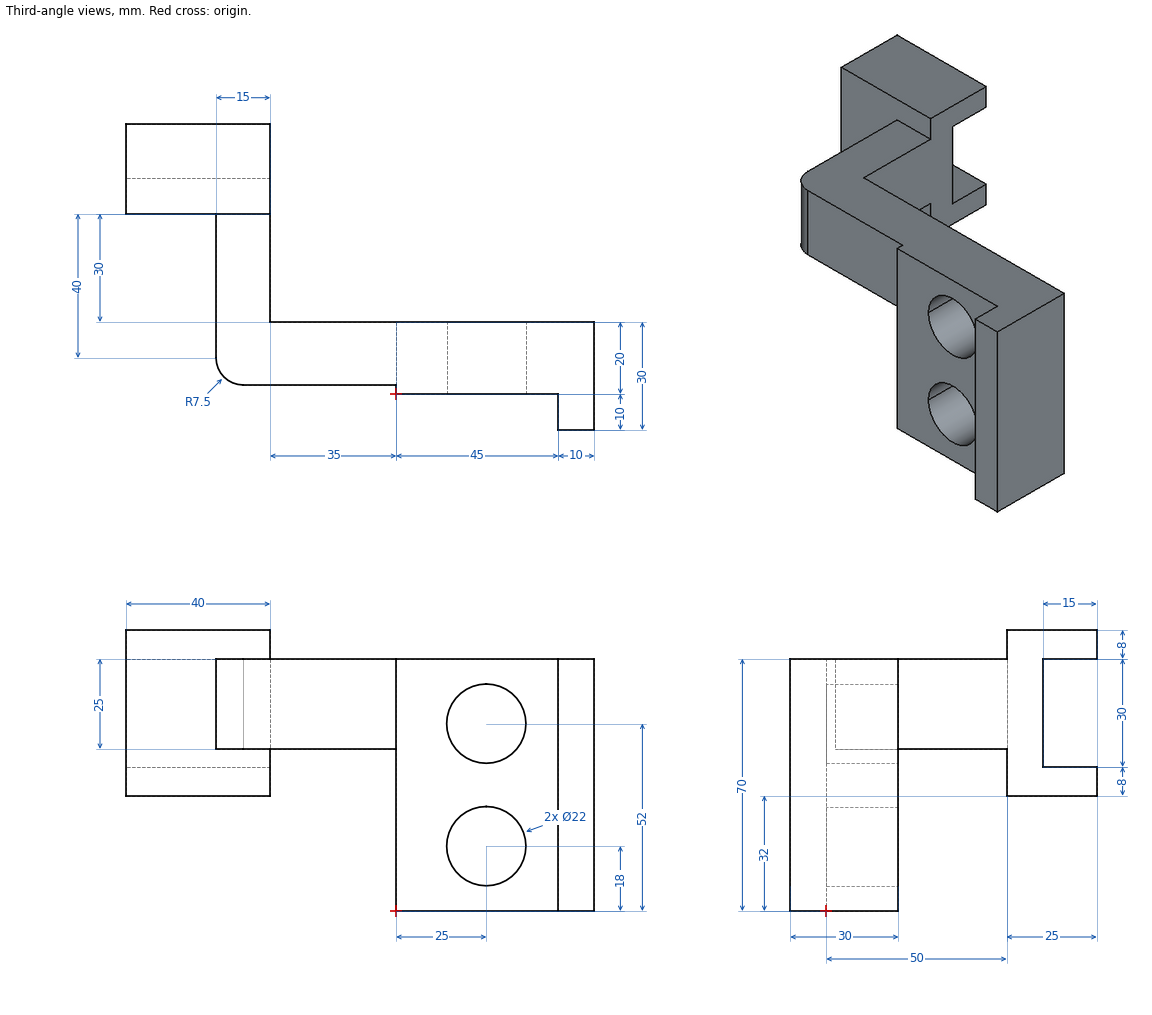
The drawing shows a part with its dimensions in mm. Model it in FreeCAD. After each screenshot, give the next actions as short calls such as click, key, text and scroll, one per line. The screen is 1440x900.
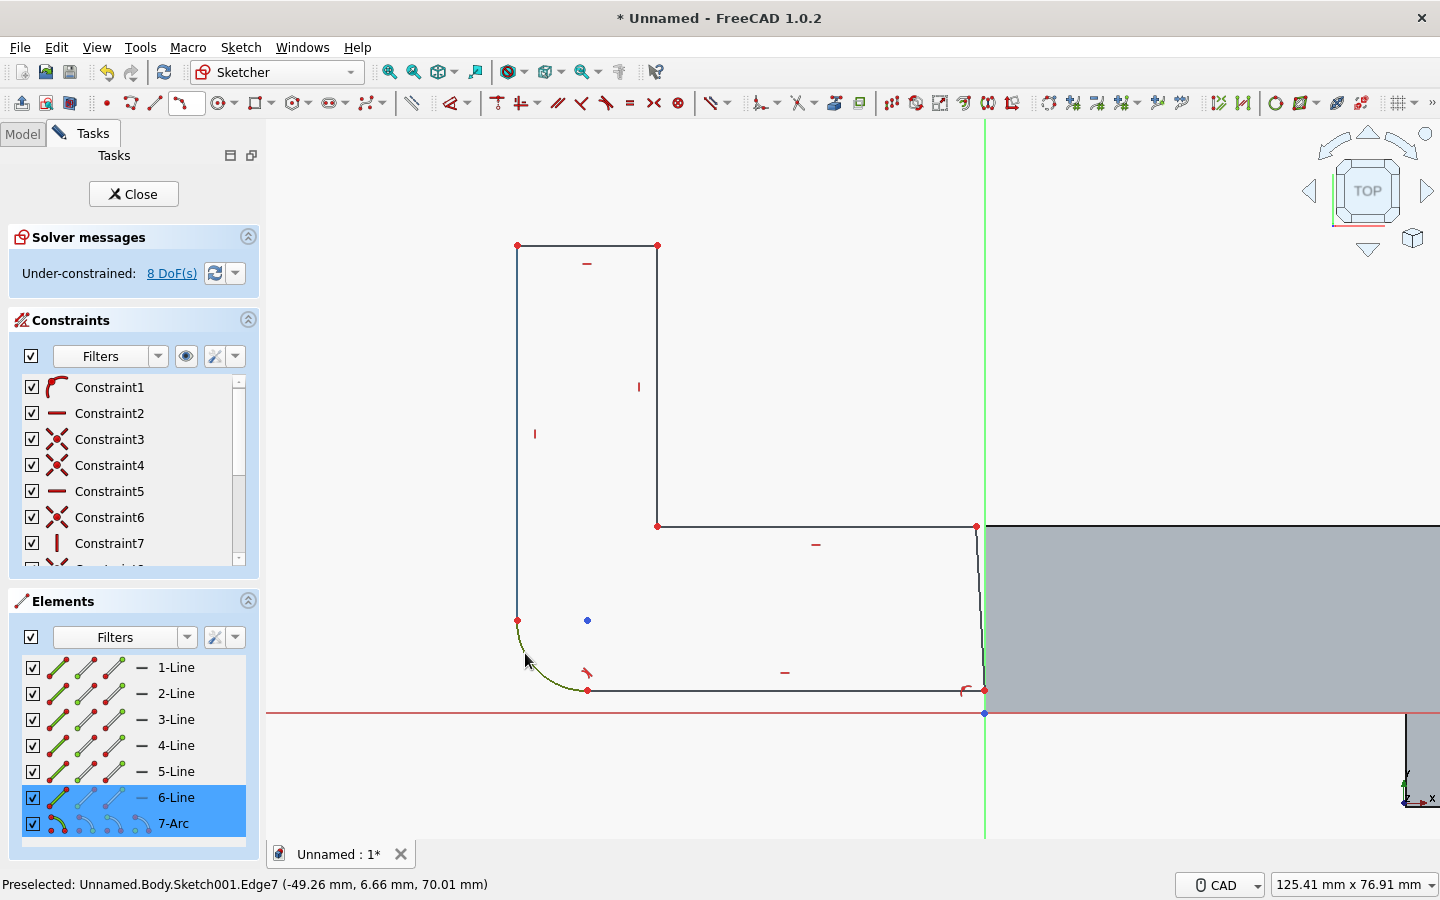
click(606, 104)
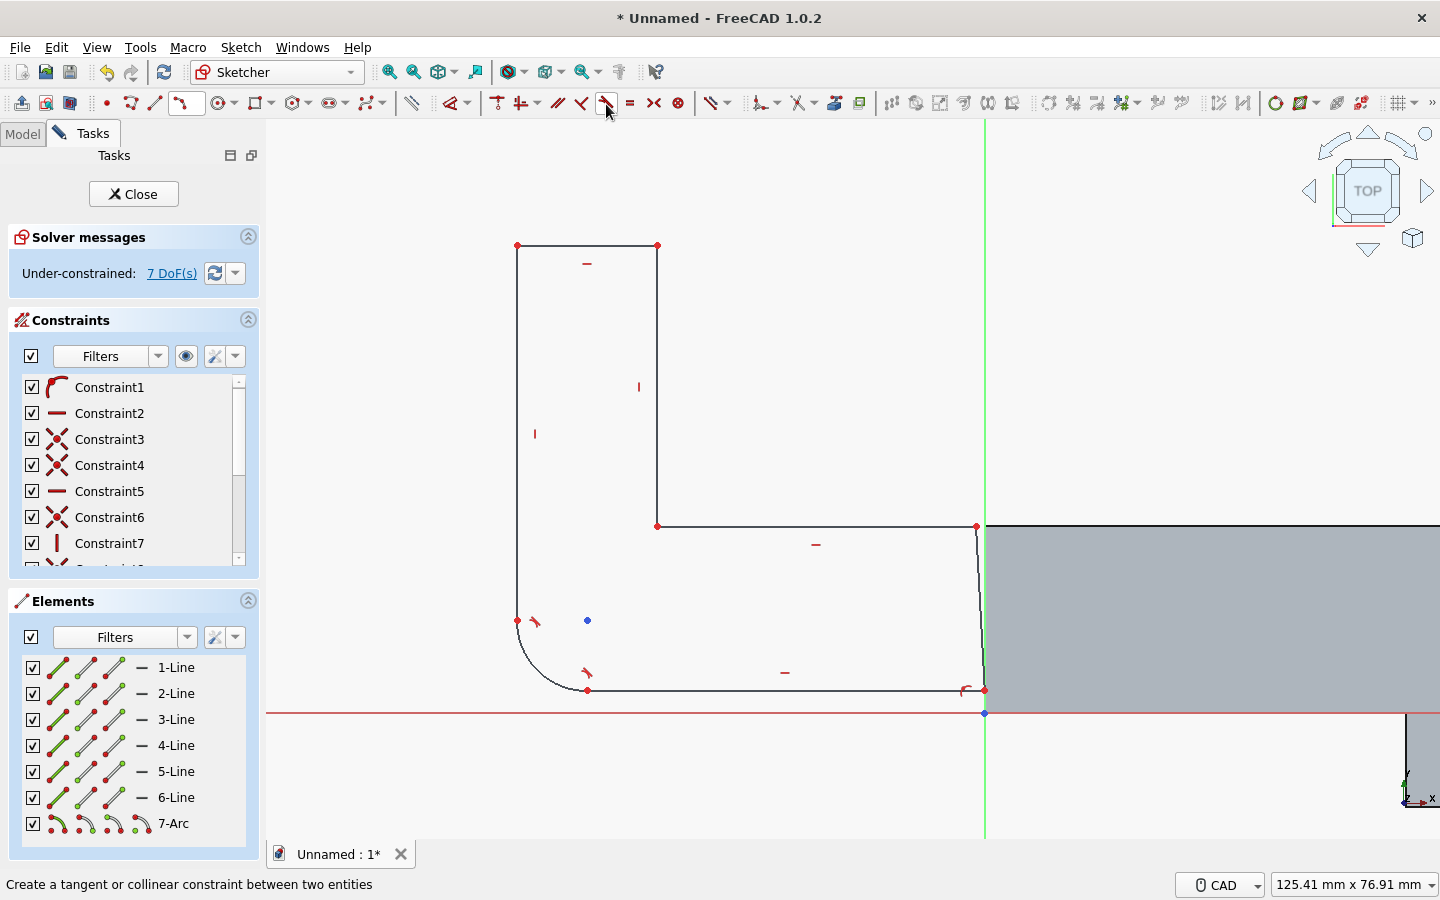
click(982, 642)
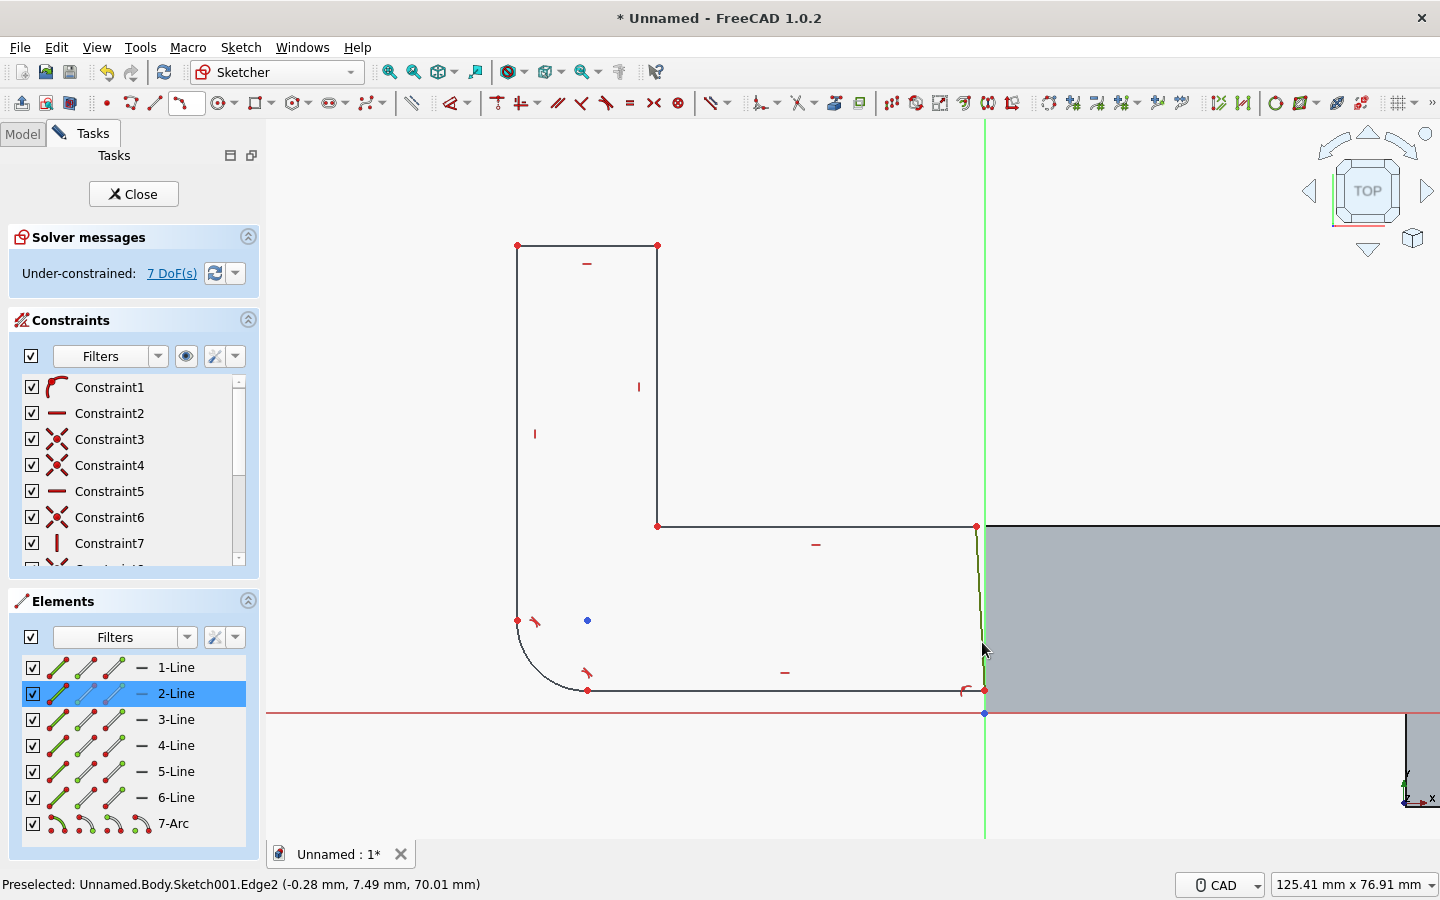
click(540, 104)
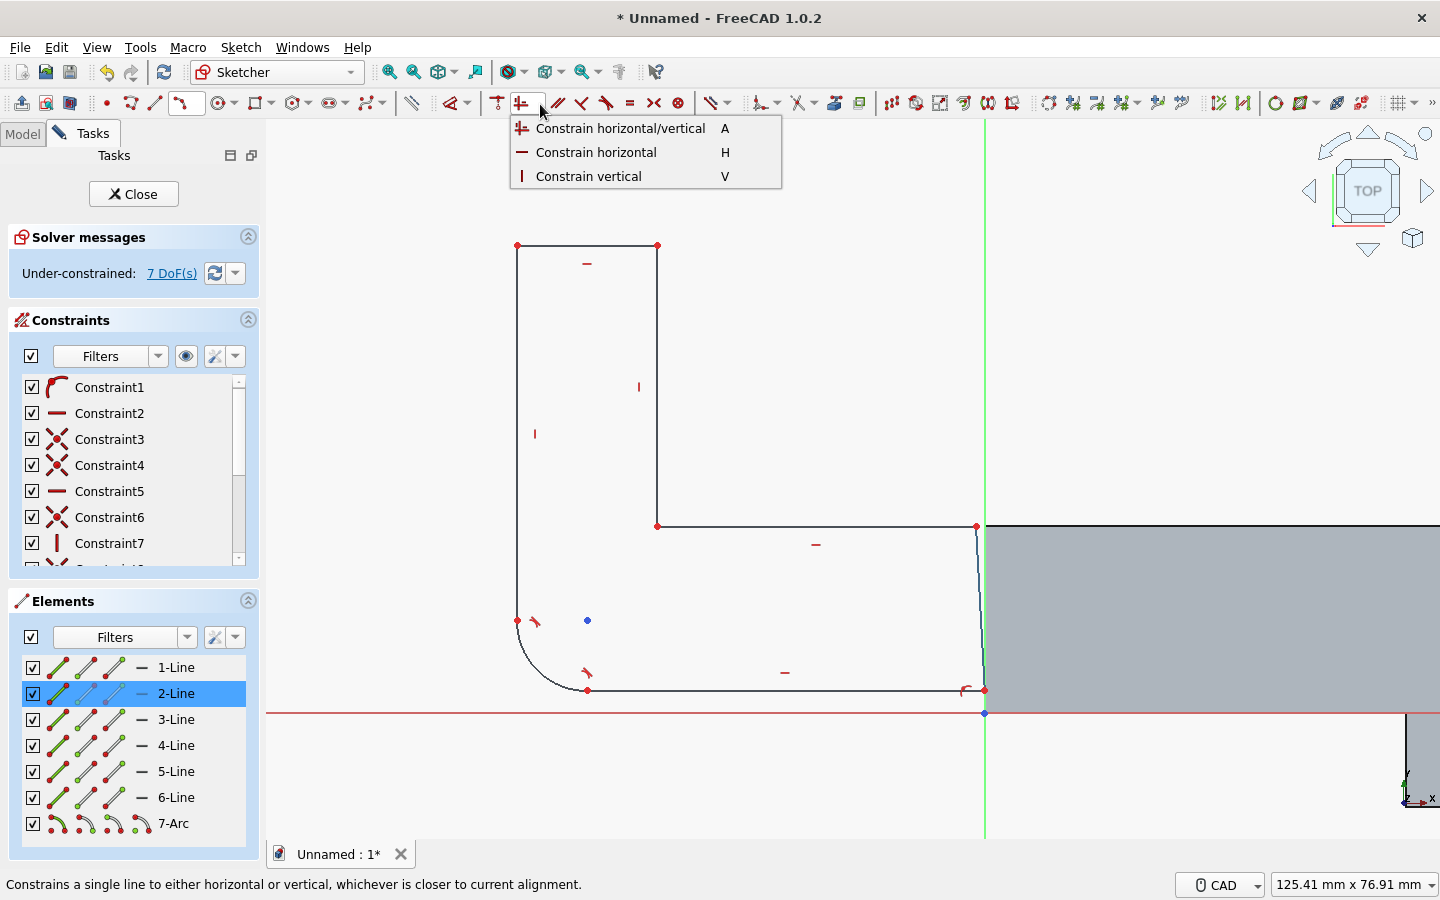
click(646, 176)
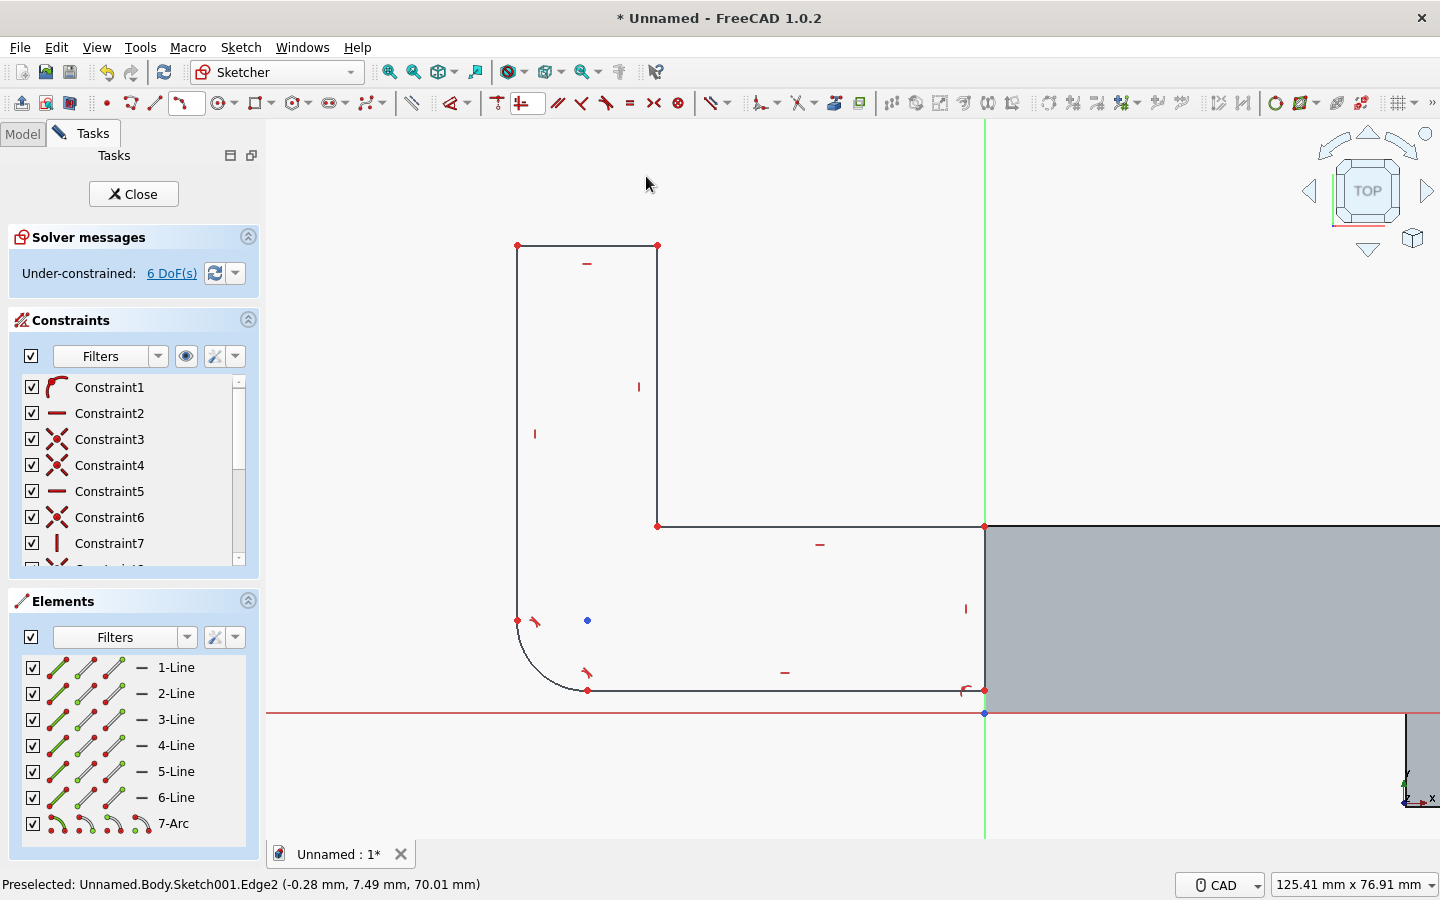
click(450, 104)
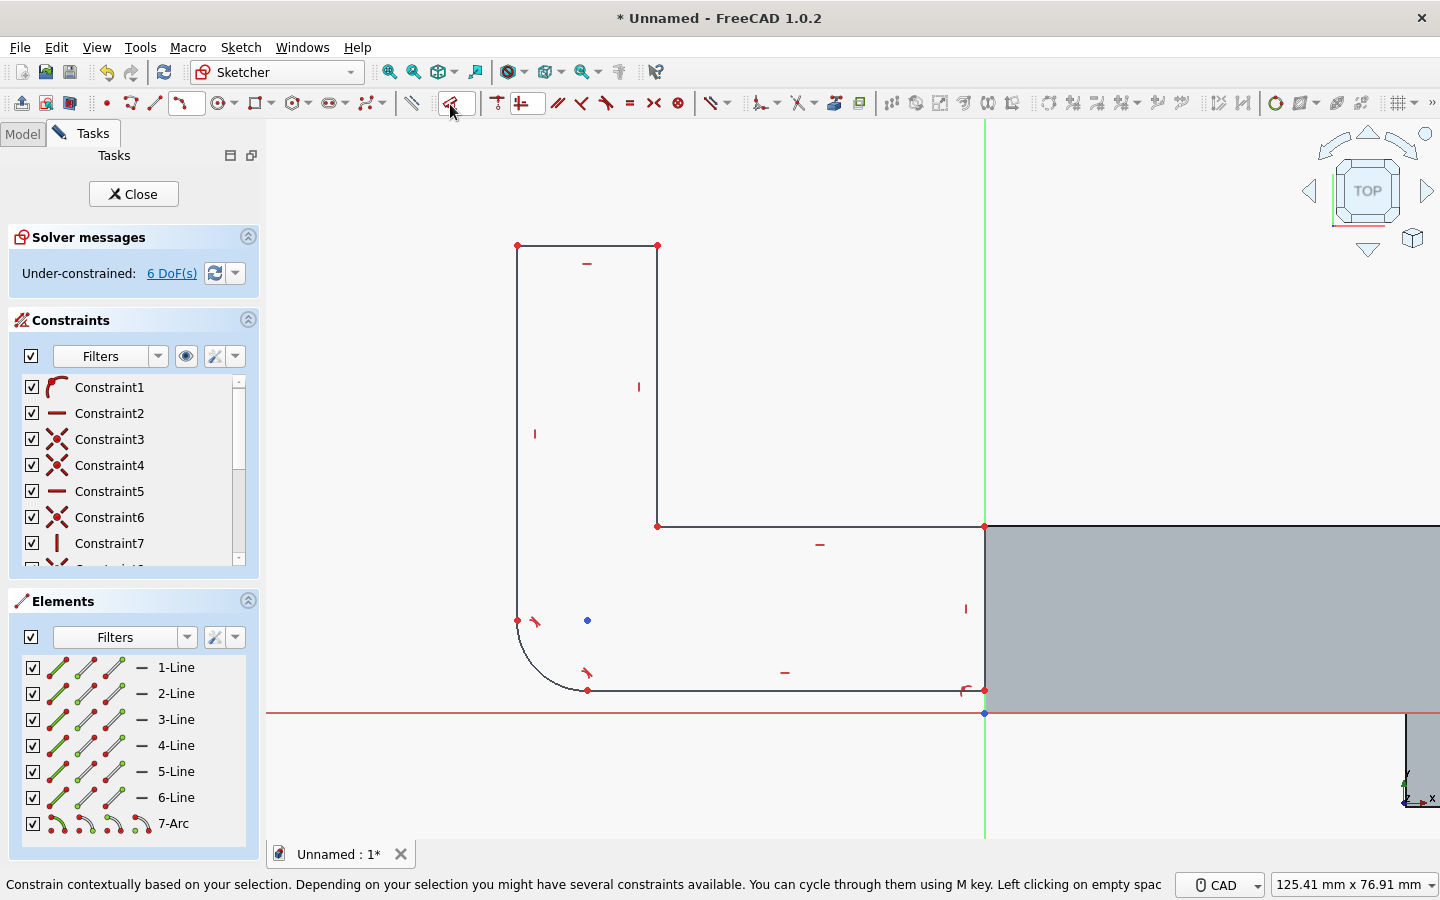
click(525, 653)
click(497, 668)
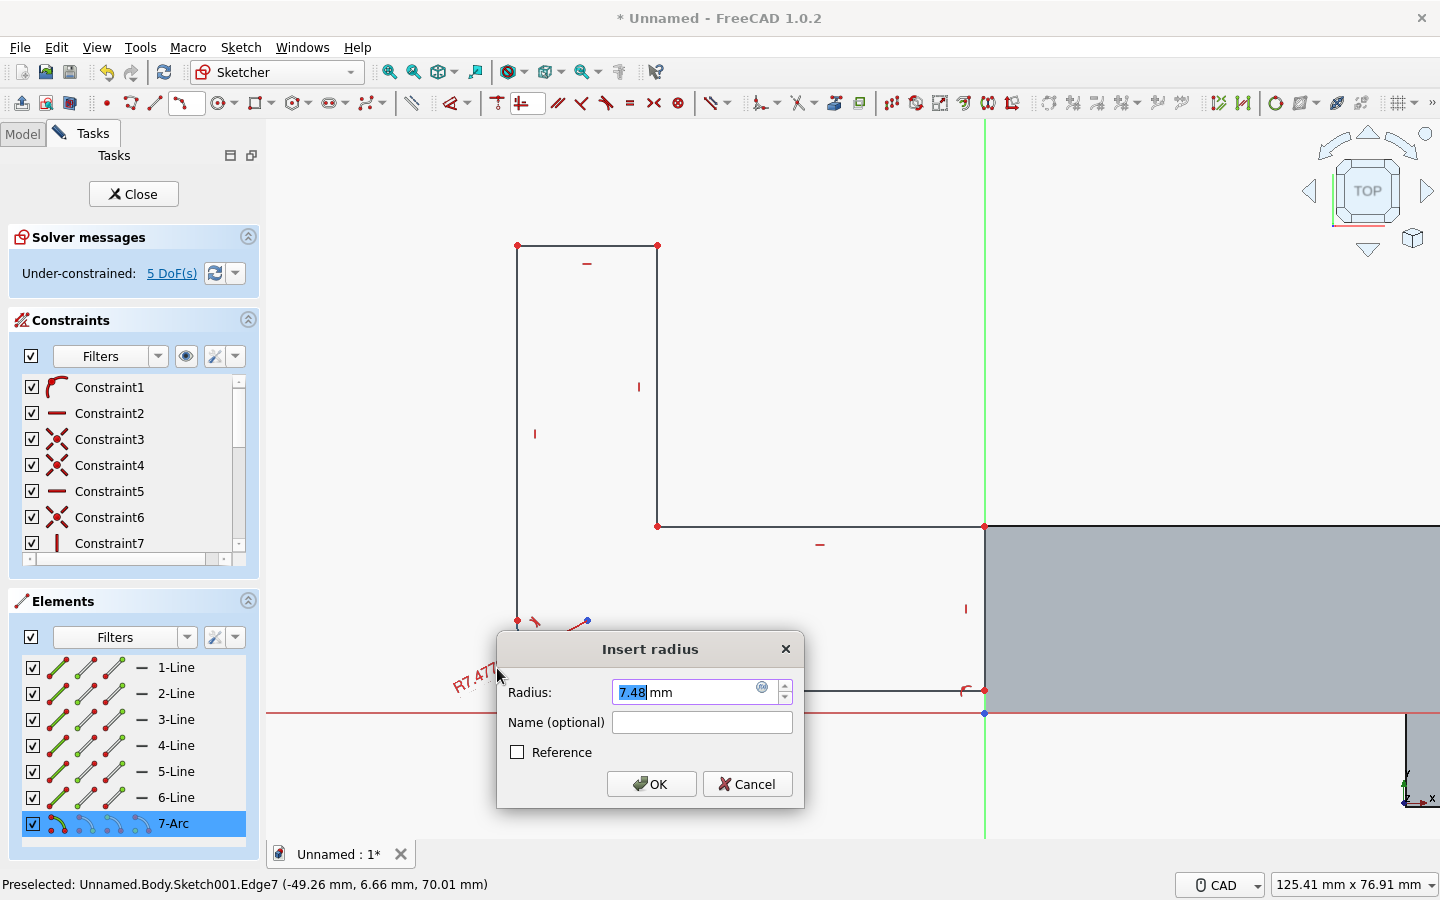
text(7.5)
key(Return)